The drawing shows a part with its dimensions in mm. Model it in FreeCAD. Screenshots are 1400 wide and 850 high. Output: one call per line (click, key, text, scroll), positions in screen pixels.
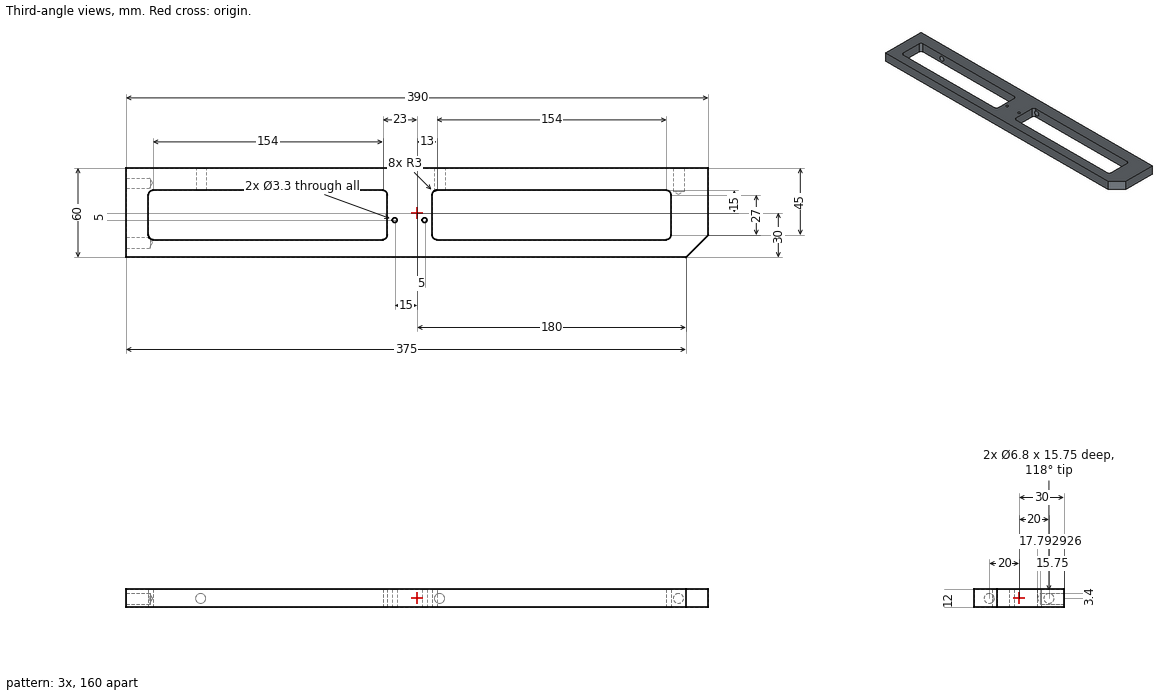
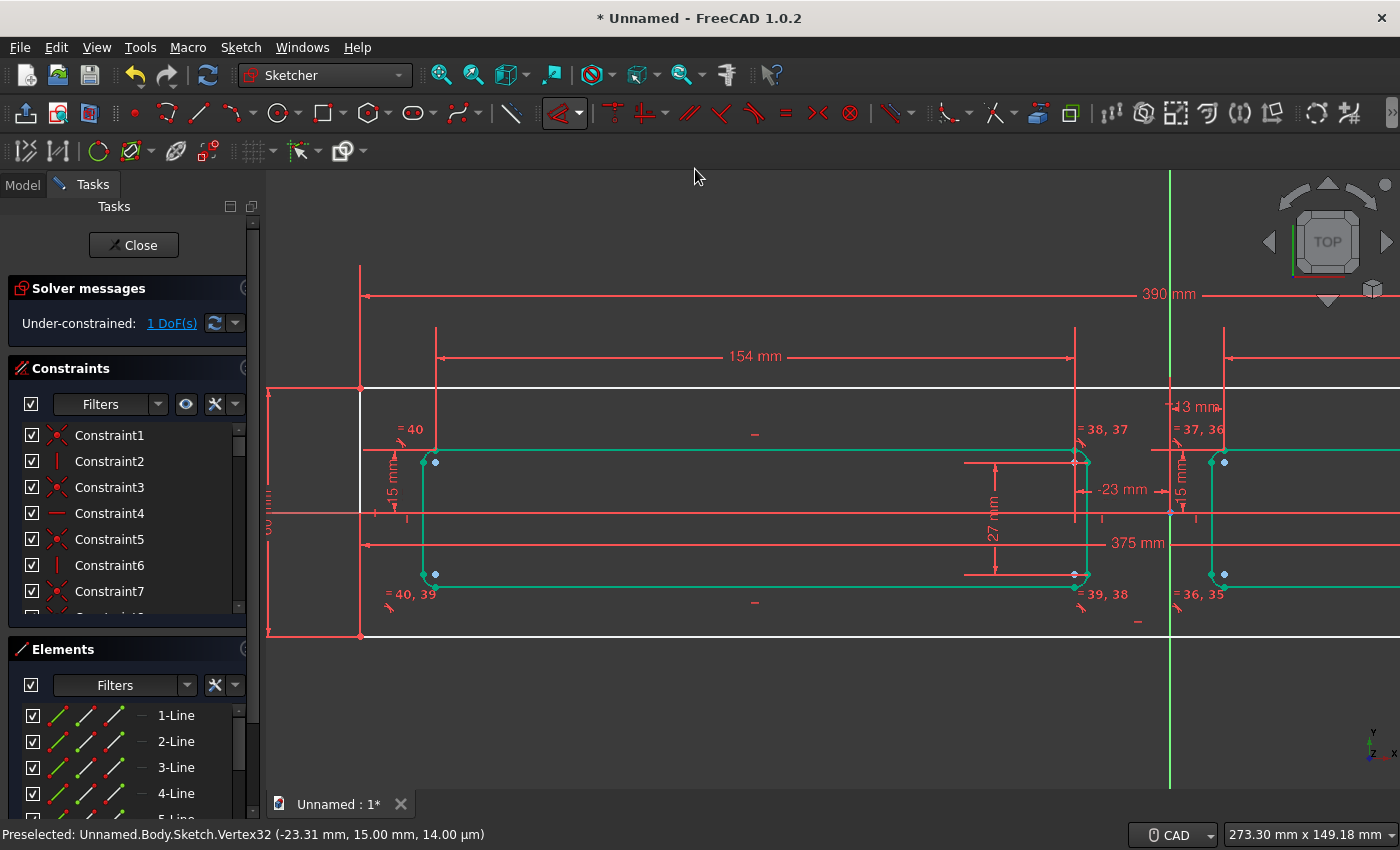
scroll(433, 453, down, 4)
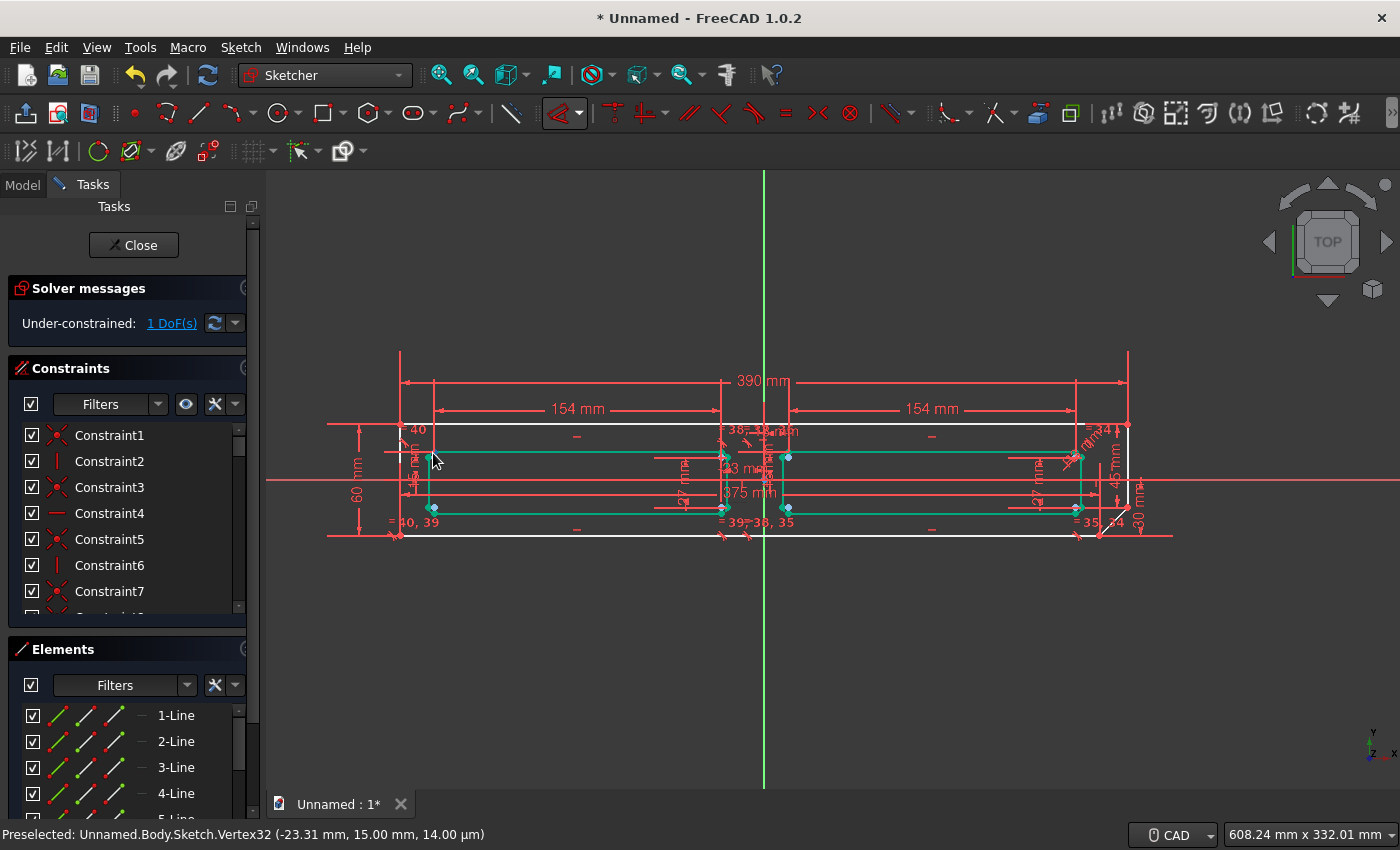
click(1100, 536)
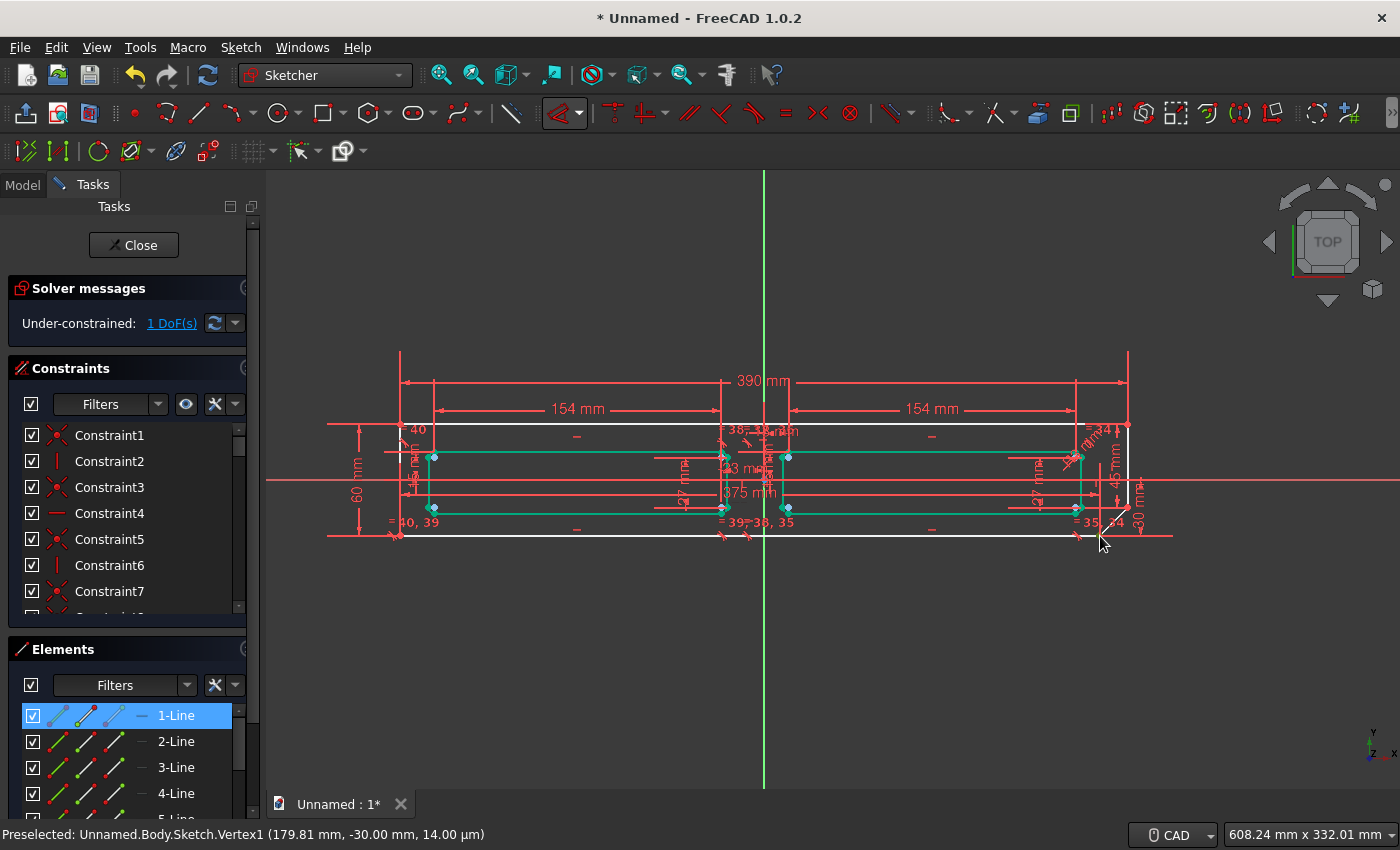
click(582, 114)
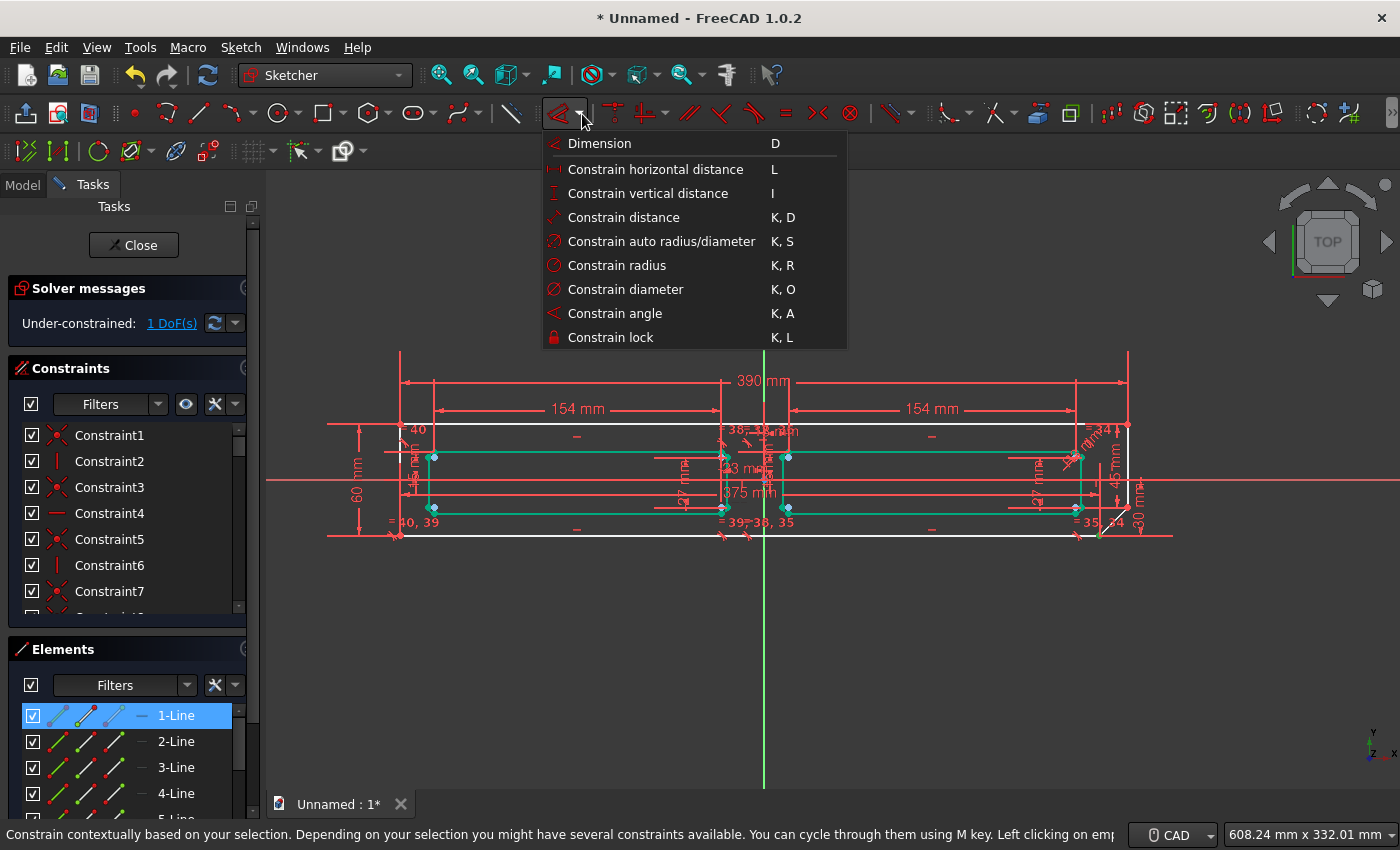
click(695, 169)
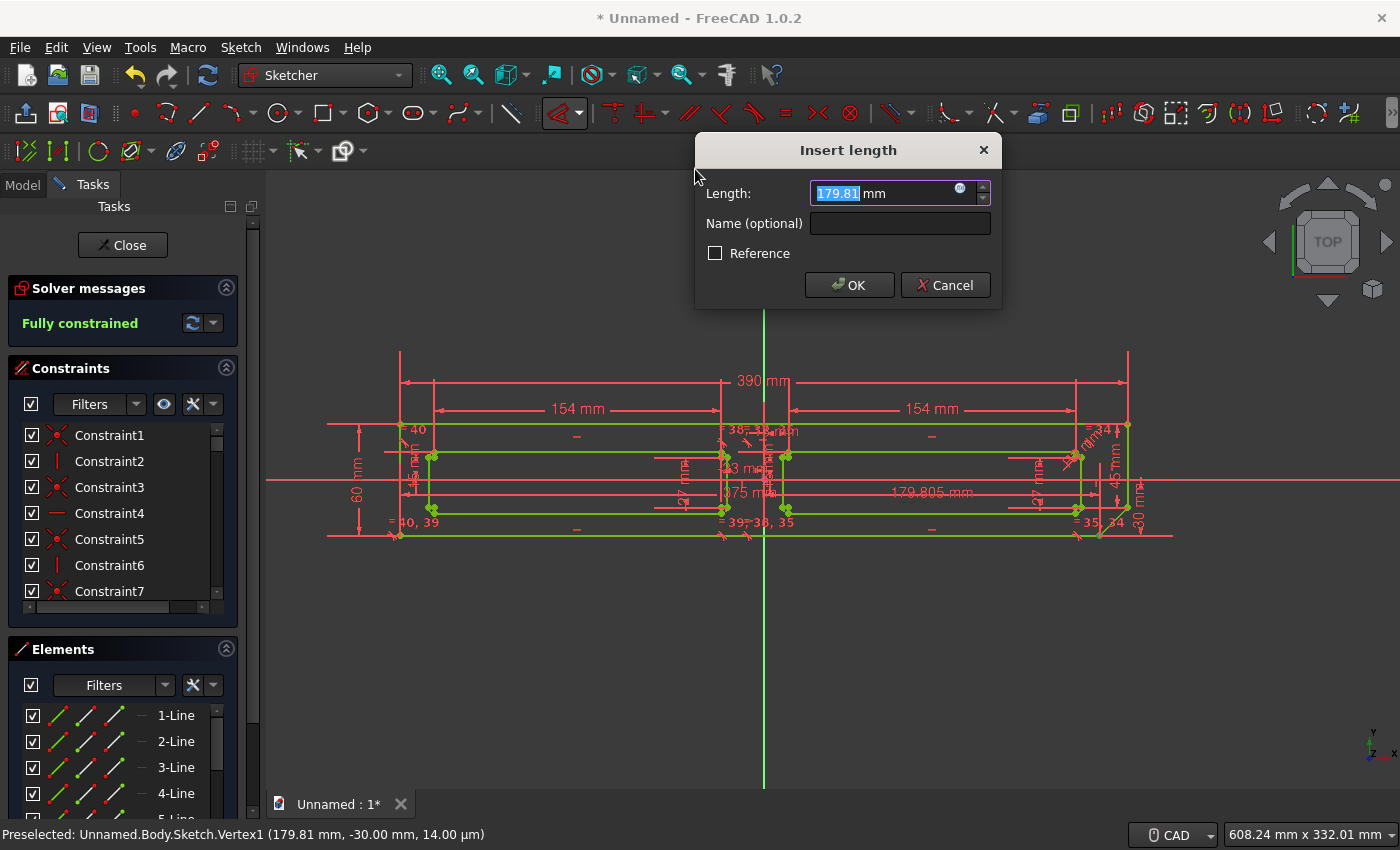
text(180)
key(Return)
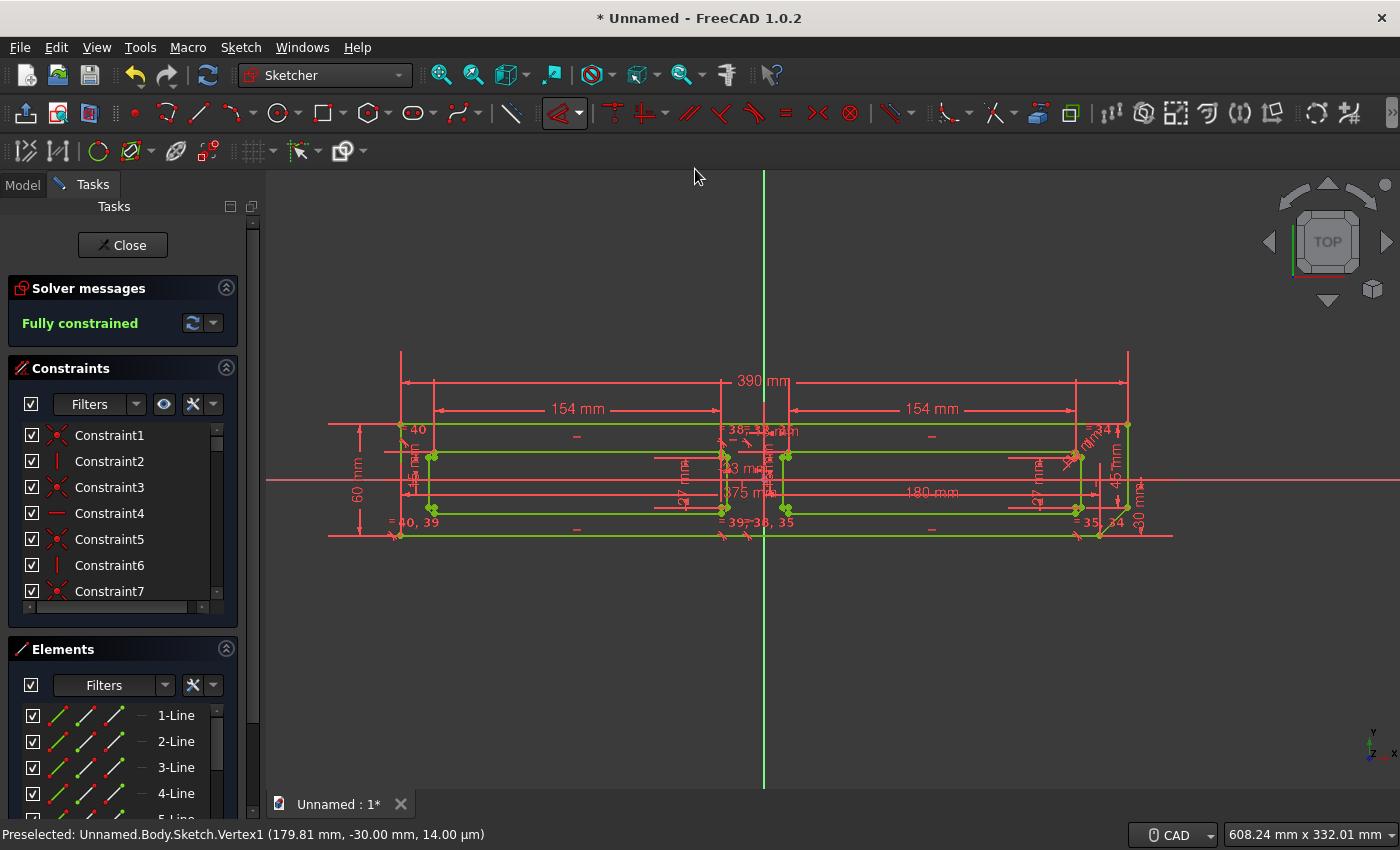
click(123, 245)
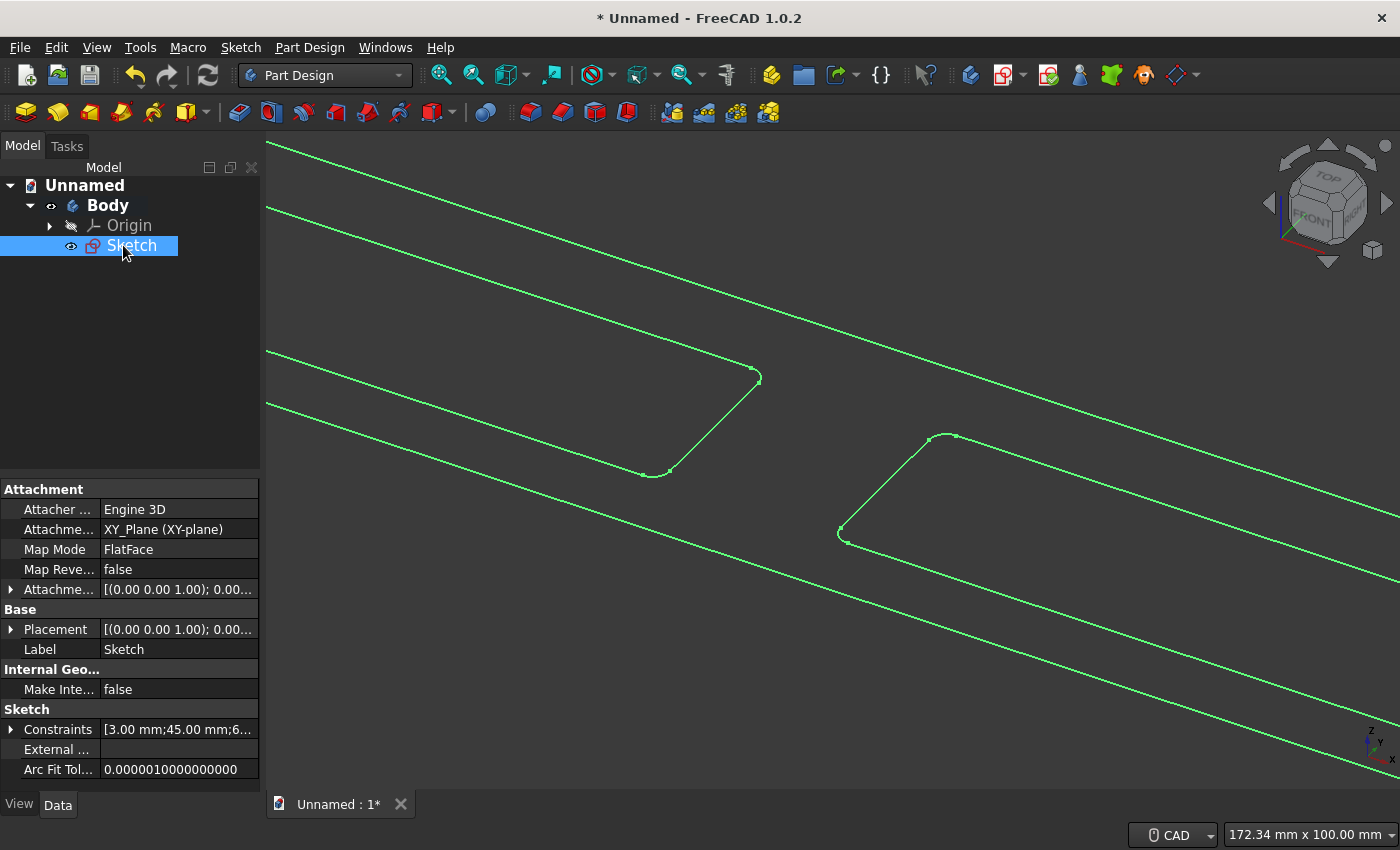
click(26, 112)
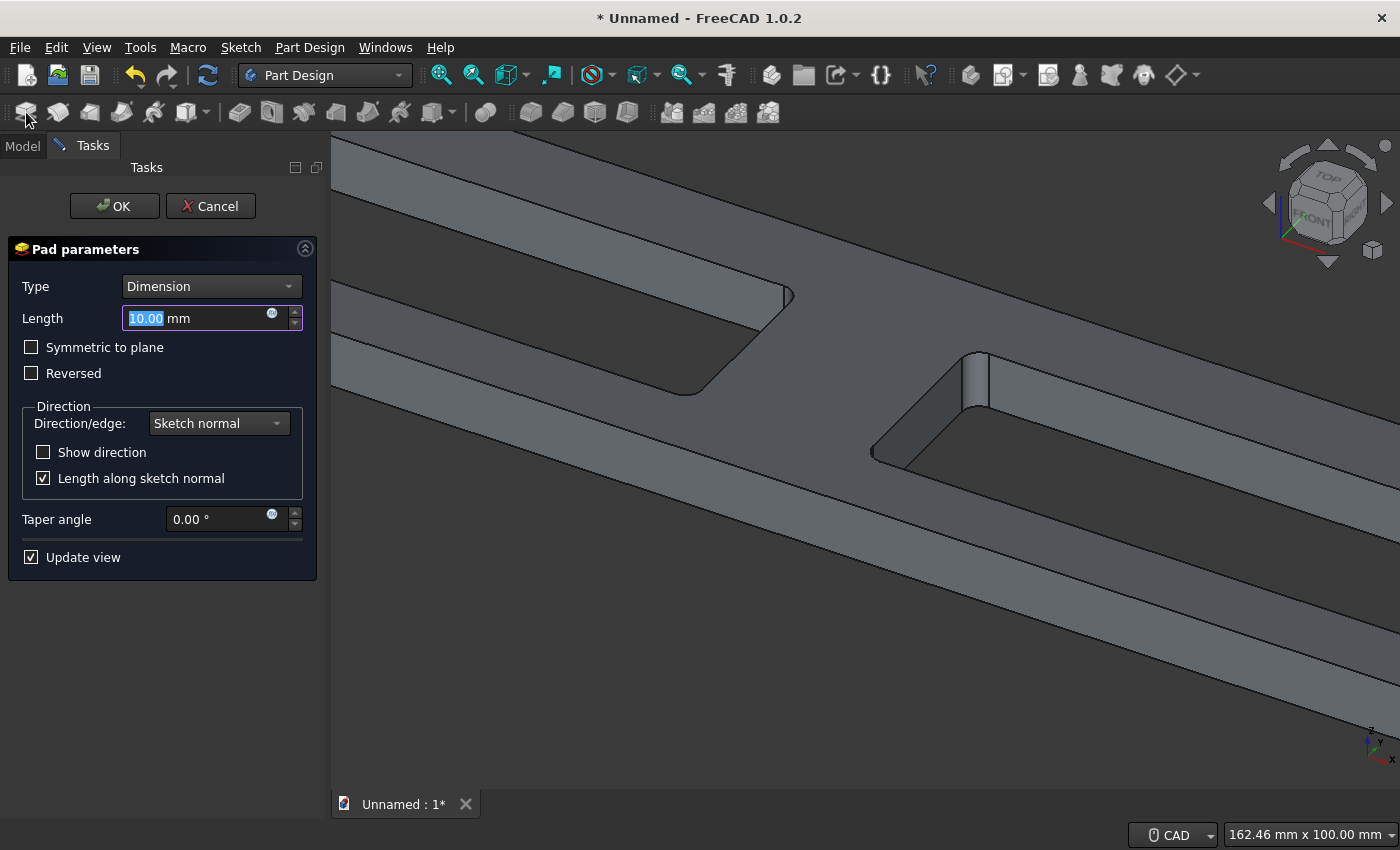
text(12)
key(Tab)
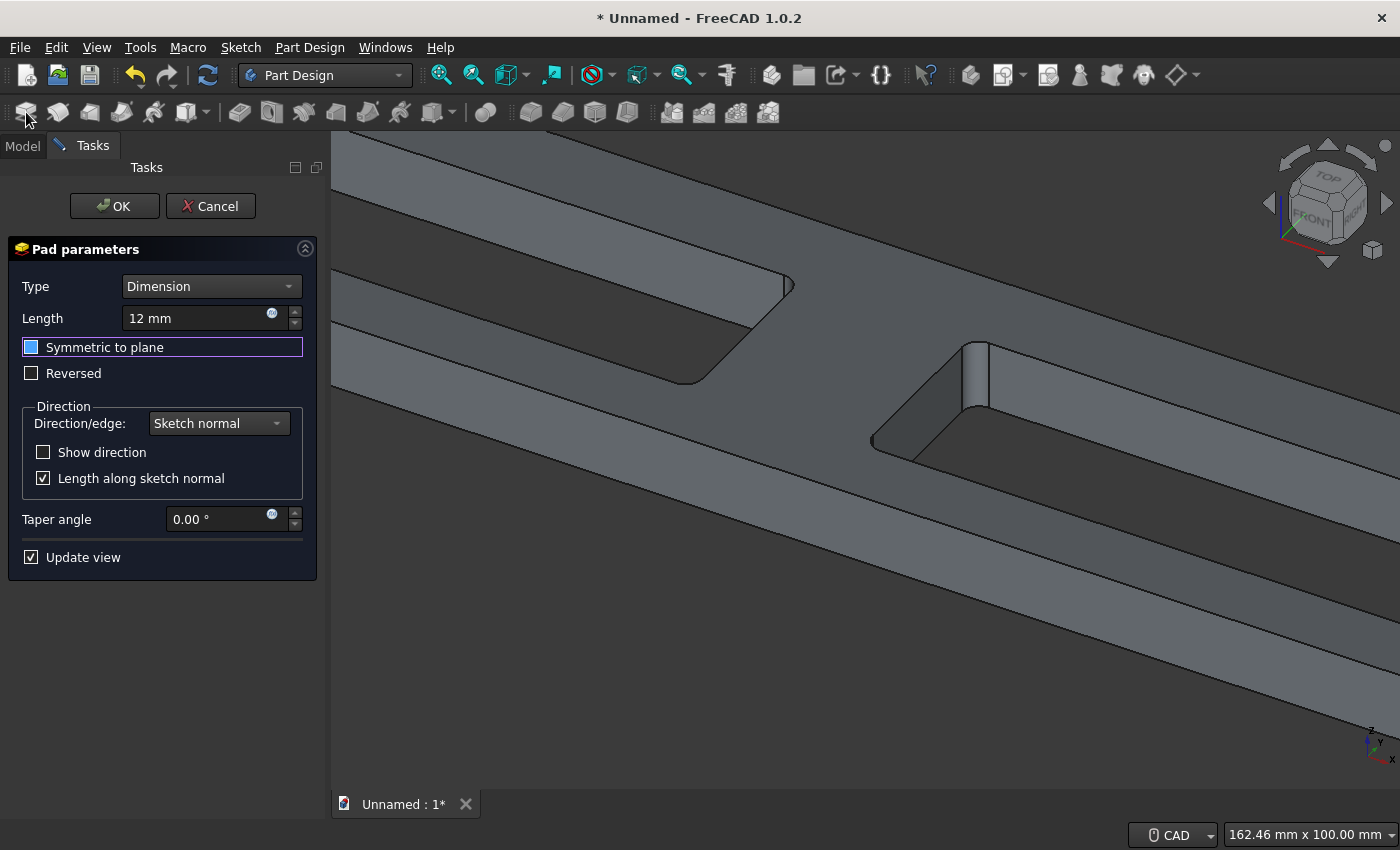
click(30, 347)